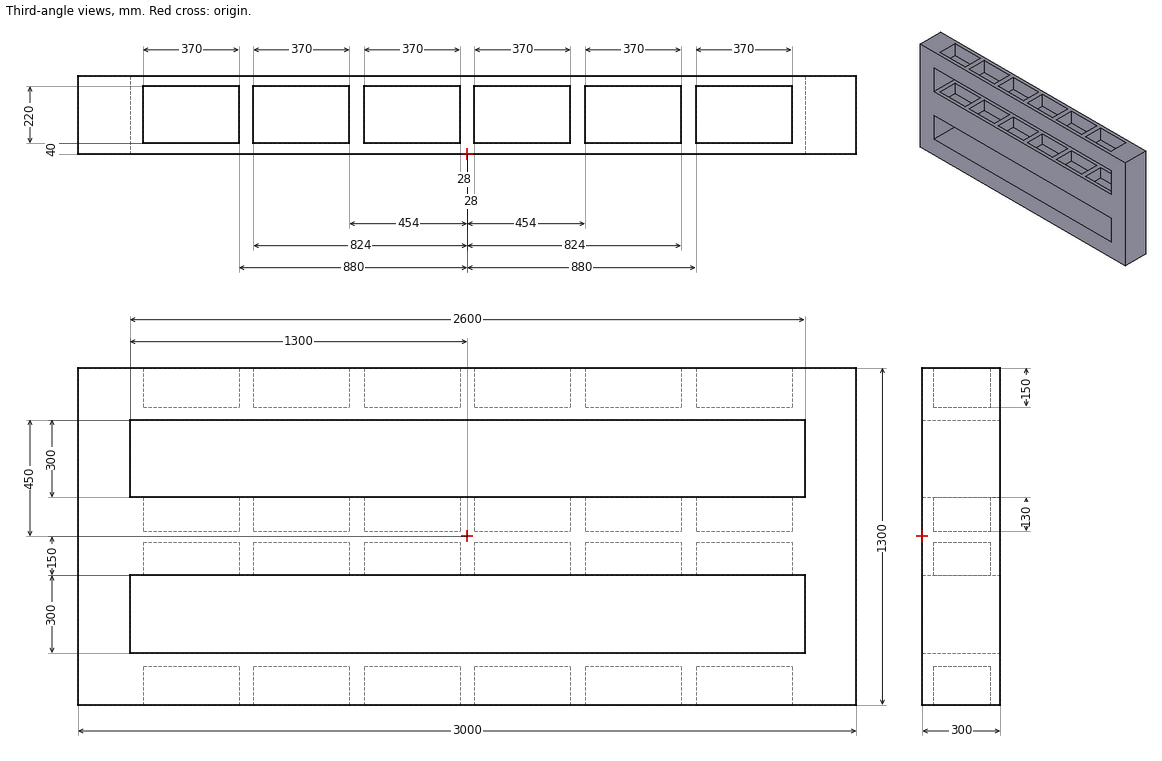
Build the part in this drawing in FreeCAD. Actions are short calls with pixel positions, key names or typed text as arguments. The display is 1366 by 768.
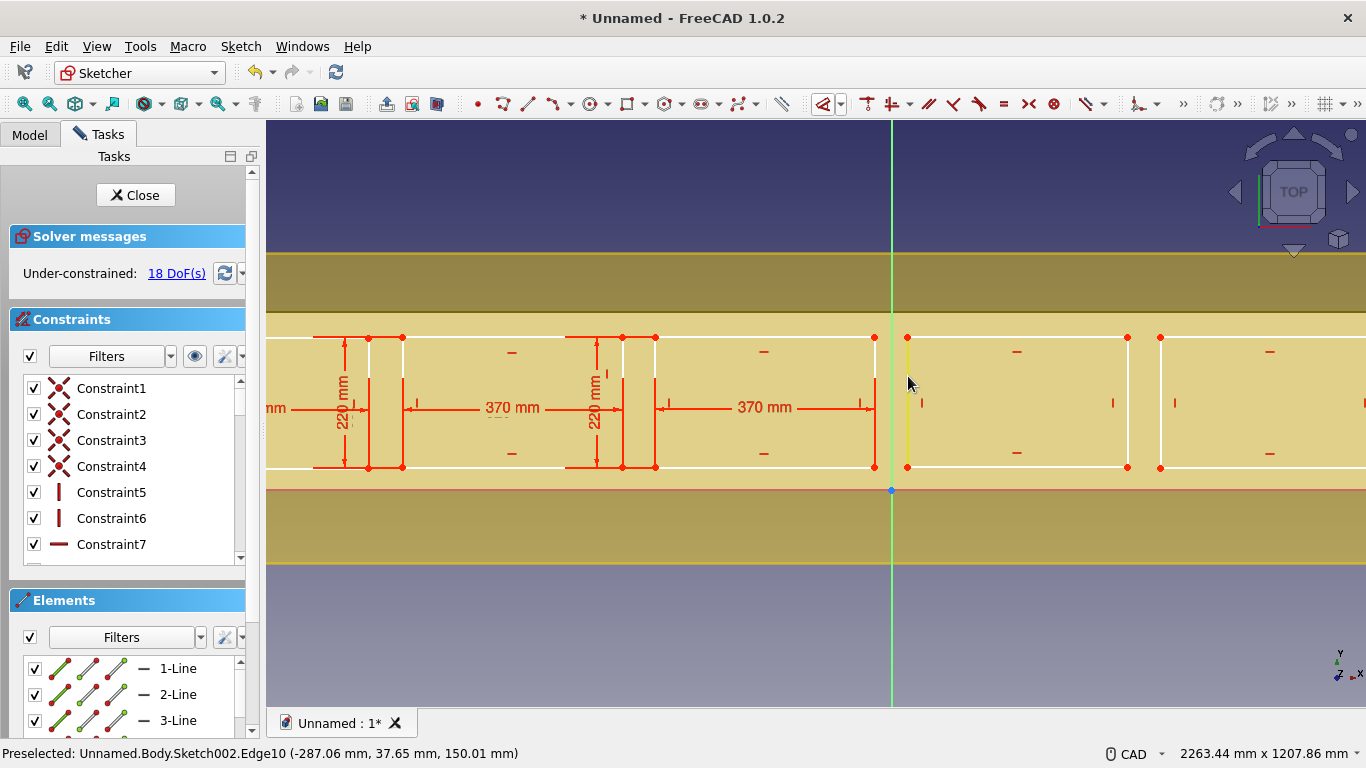
click(908, 376)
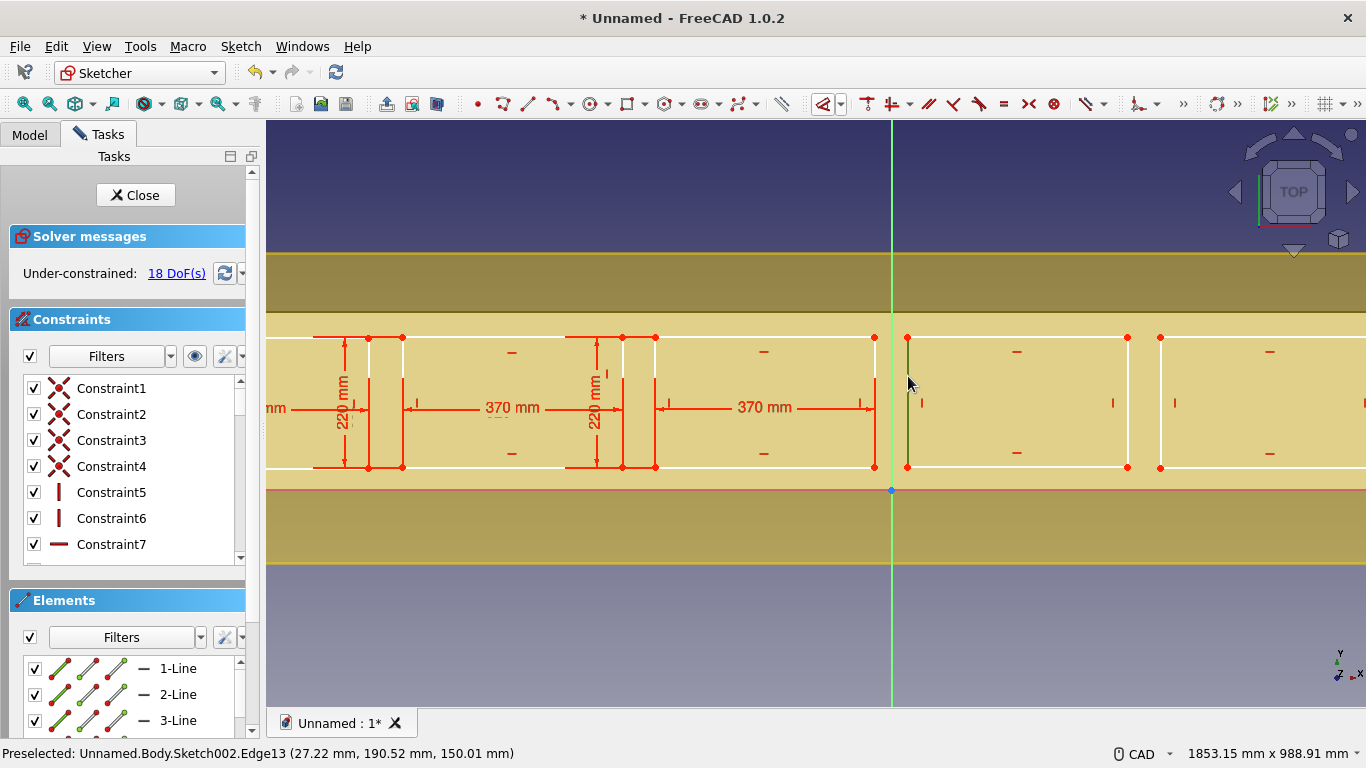
key(i)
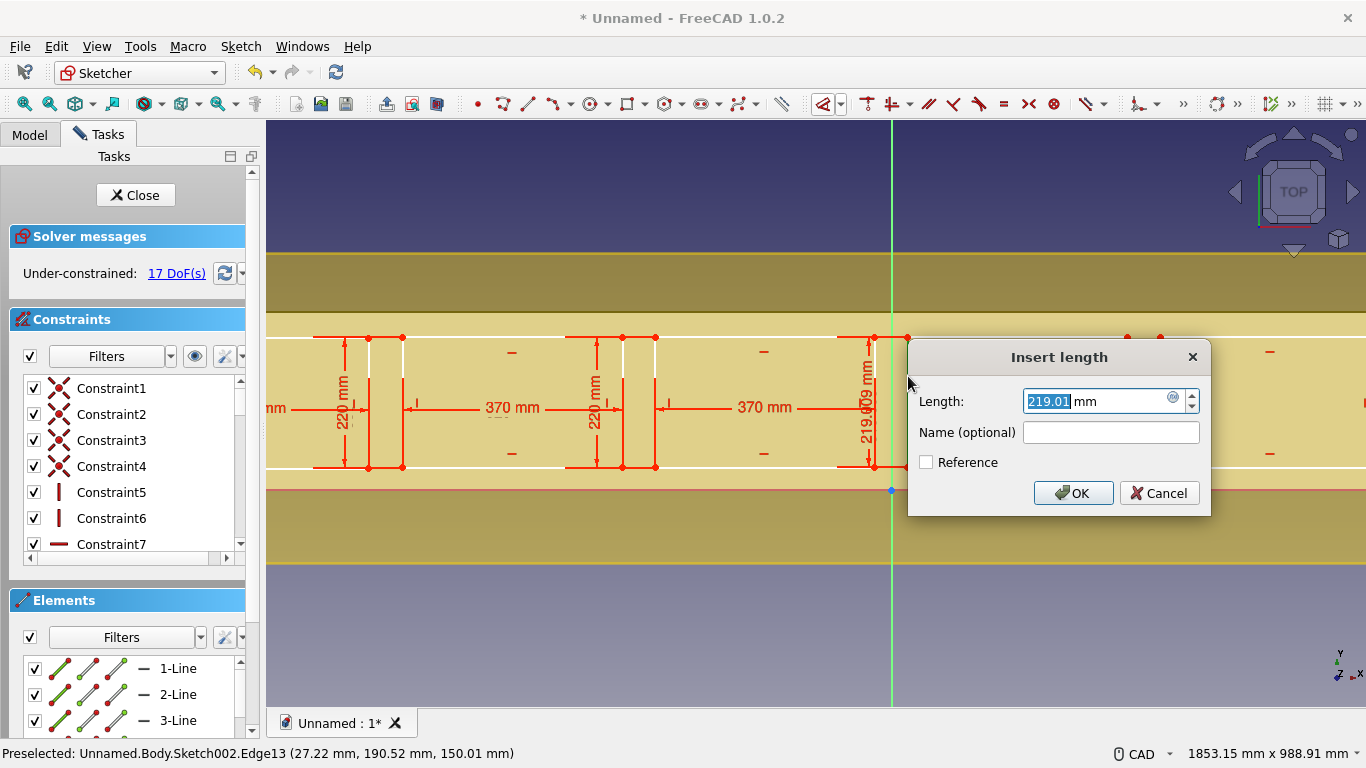
text(220)
key(Return)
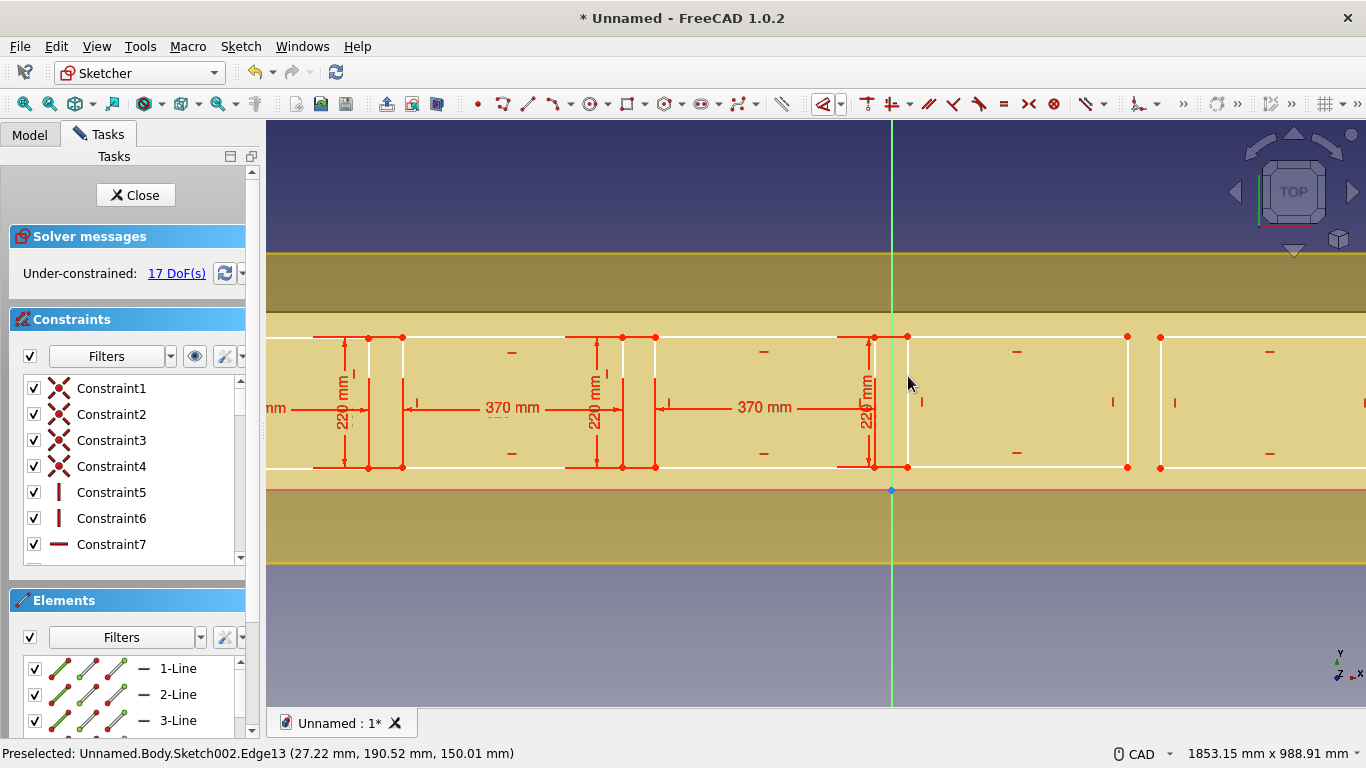
click(974, 467)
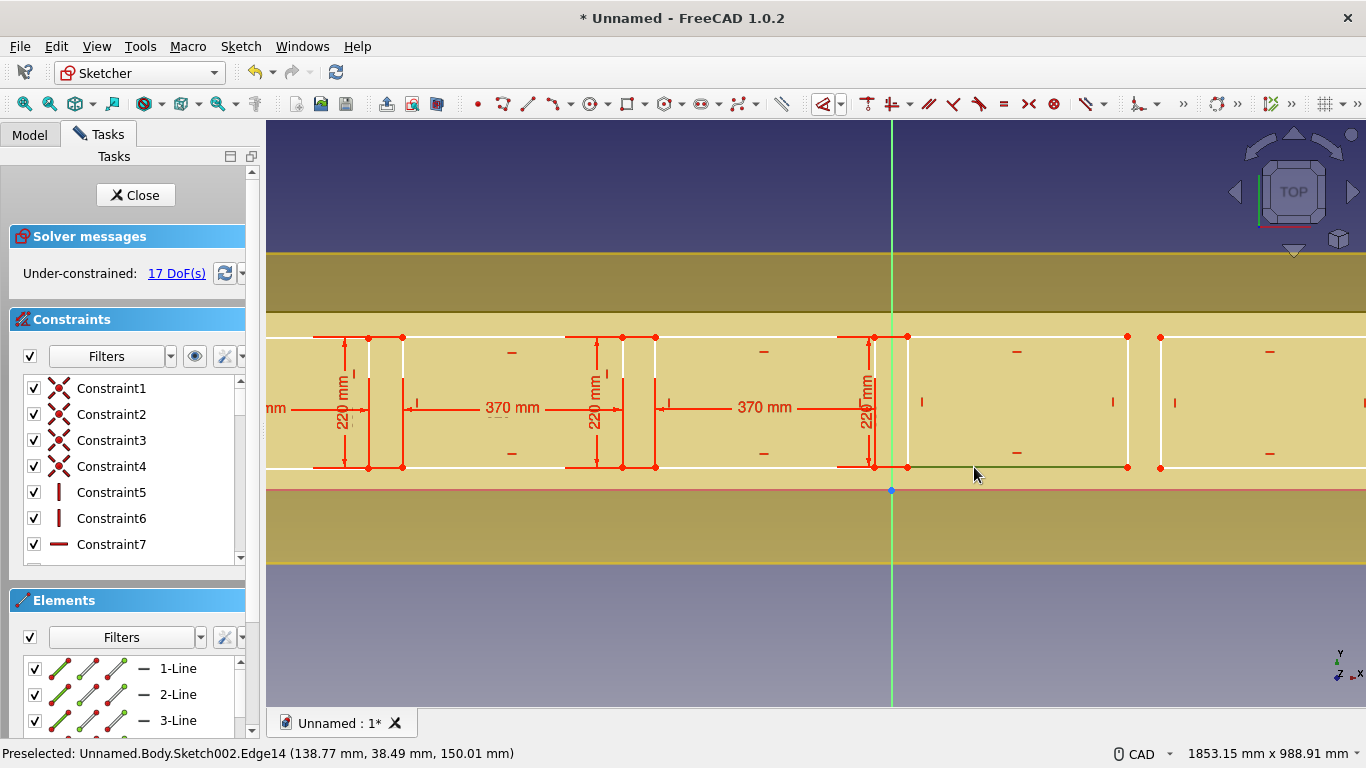
key(l)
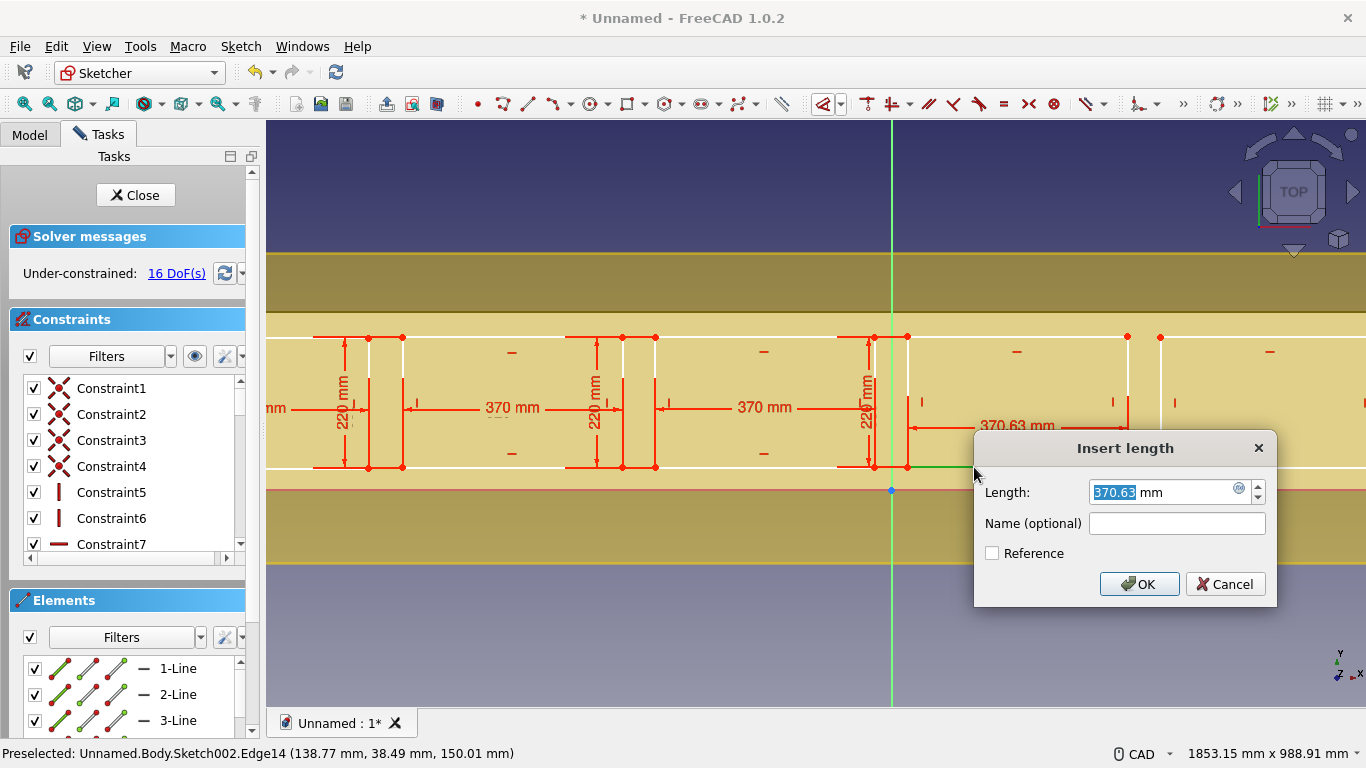
text(370)
key(Return)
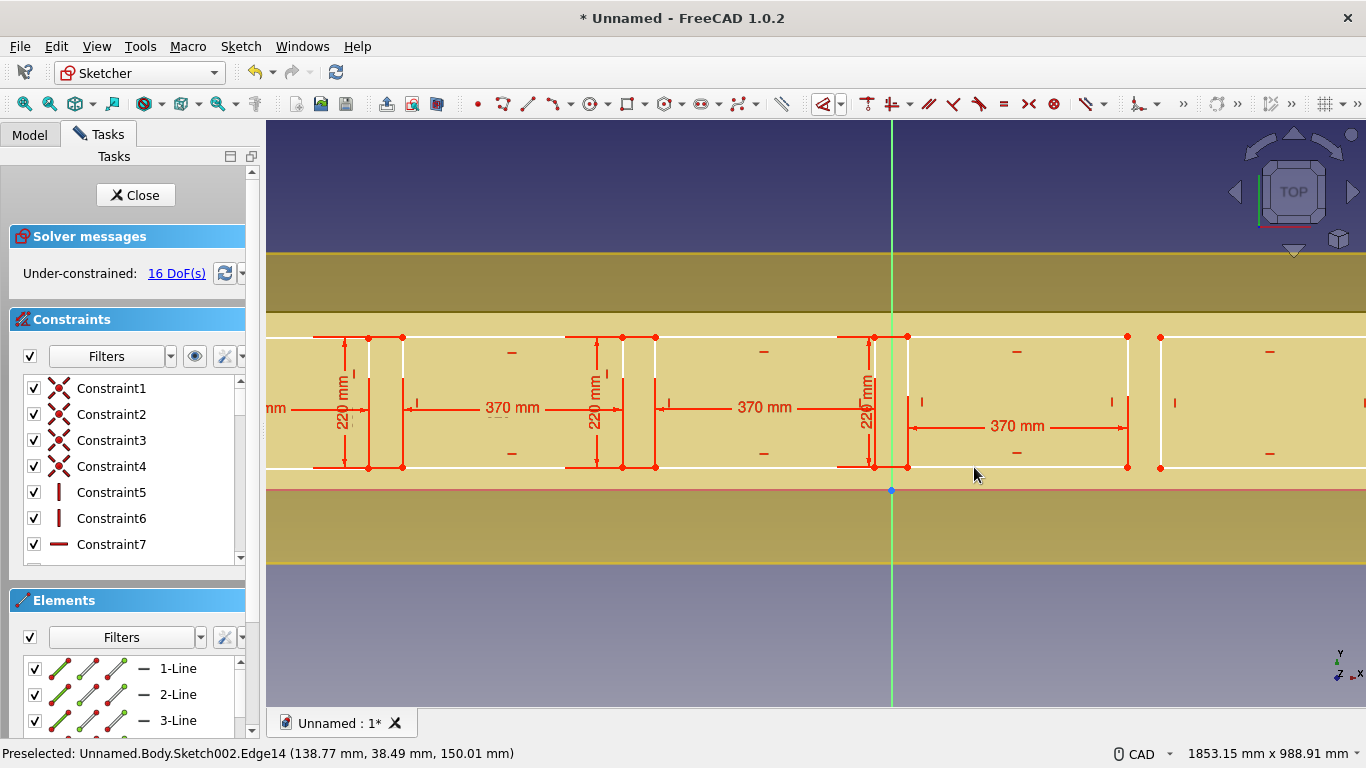
click(1161, 376)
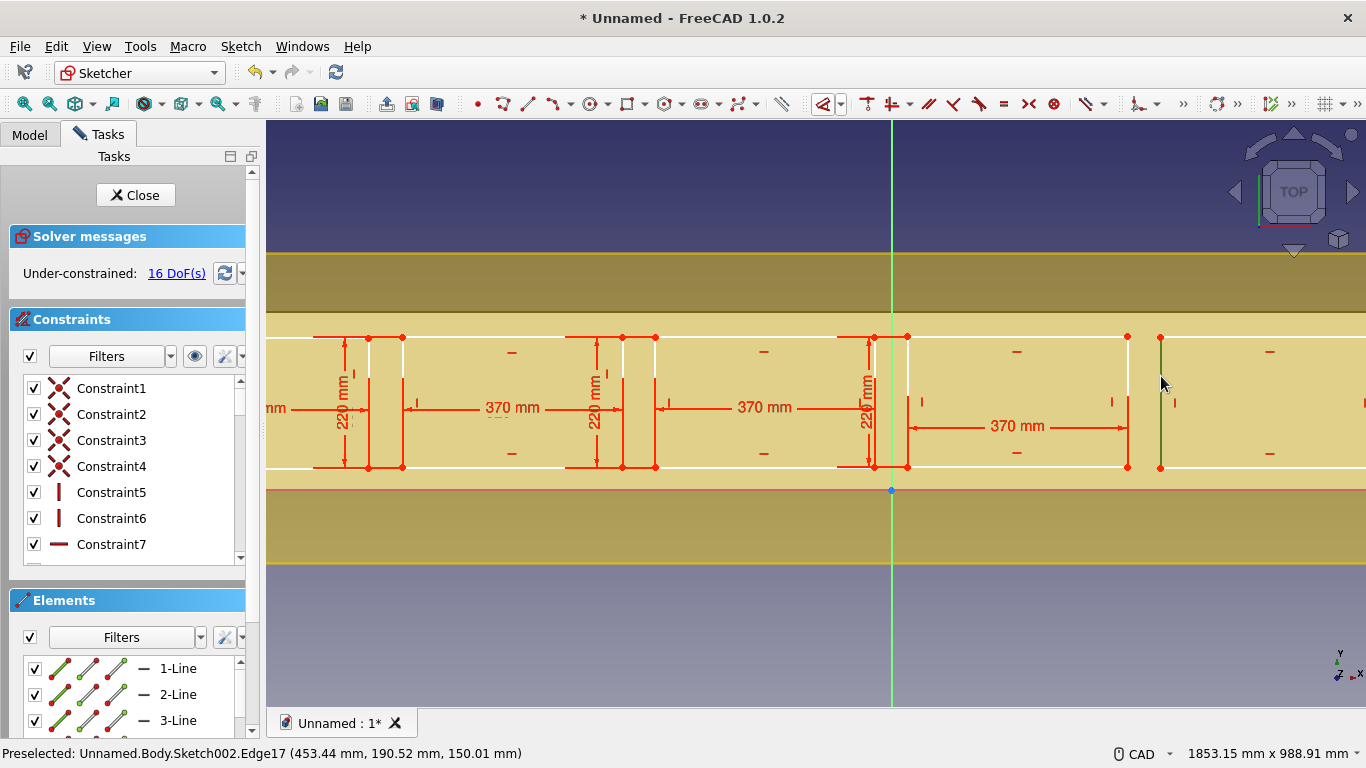
key(i)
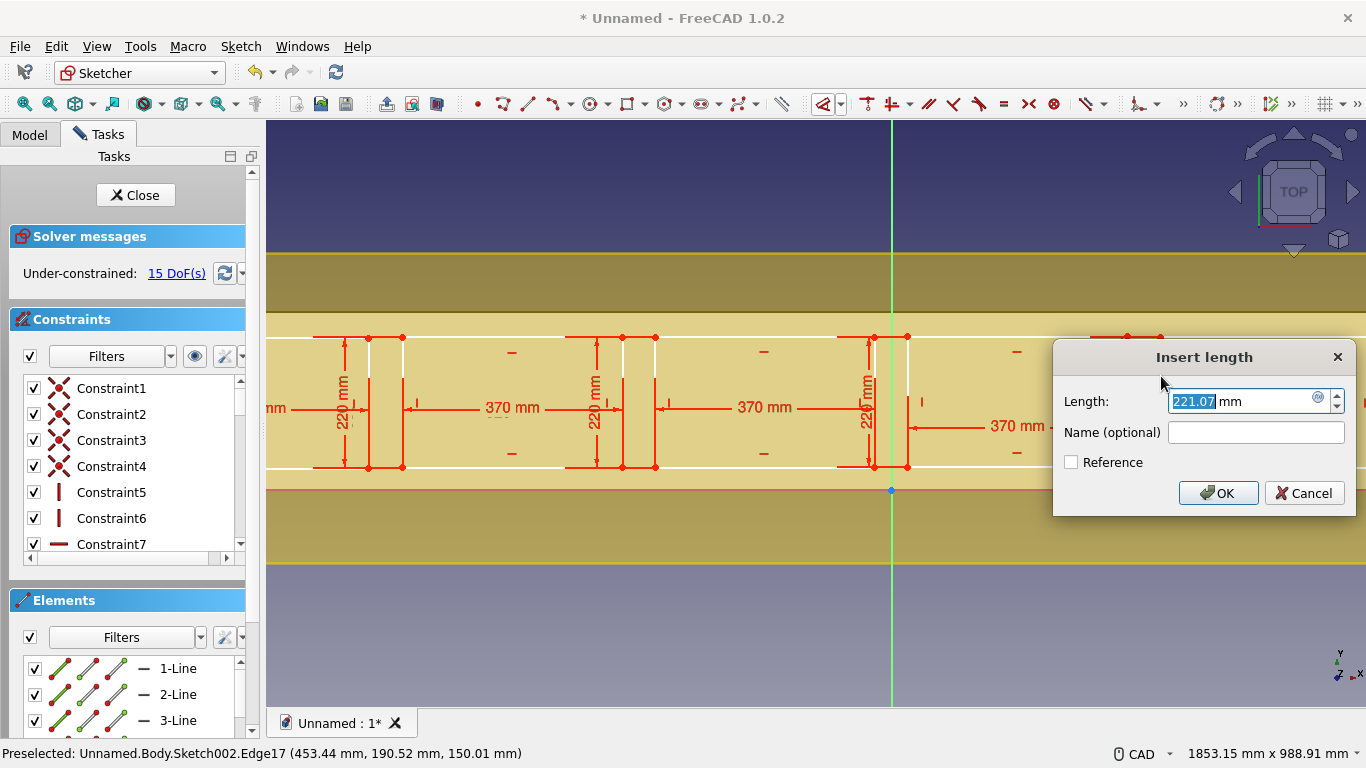
text(220)
key(Return)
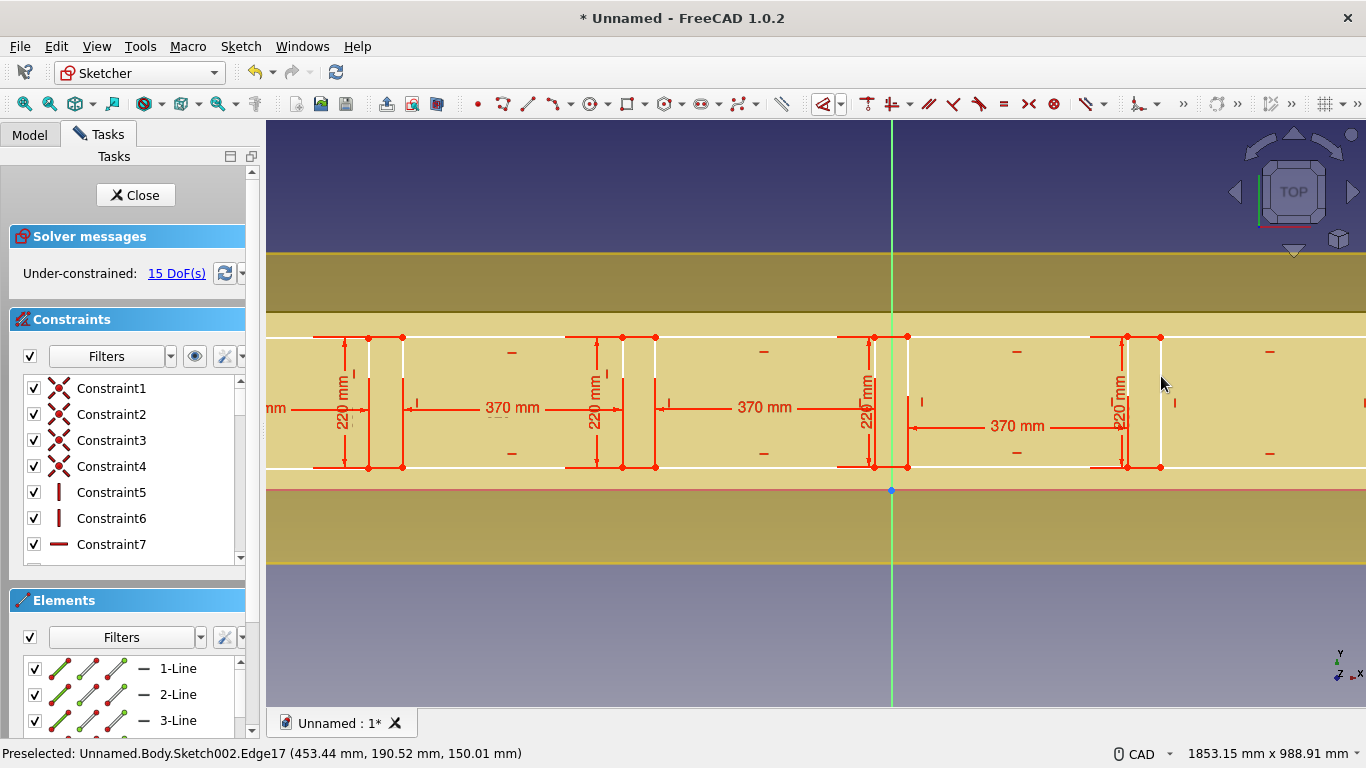
scroll(630, 414, down, 4)